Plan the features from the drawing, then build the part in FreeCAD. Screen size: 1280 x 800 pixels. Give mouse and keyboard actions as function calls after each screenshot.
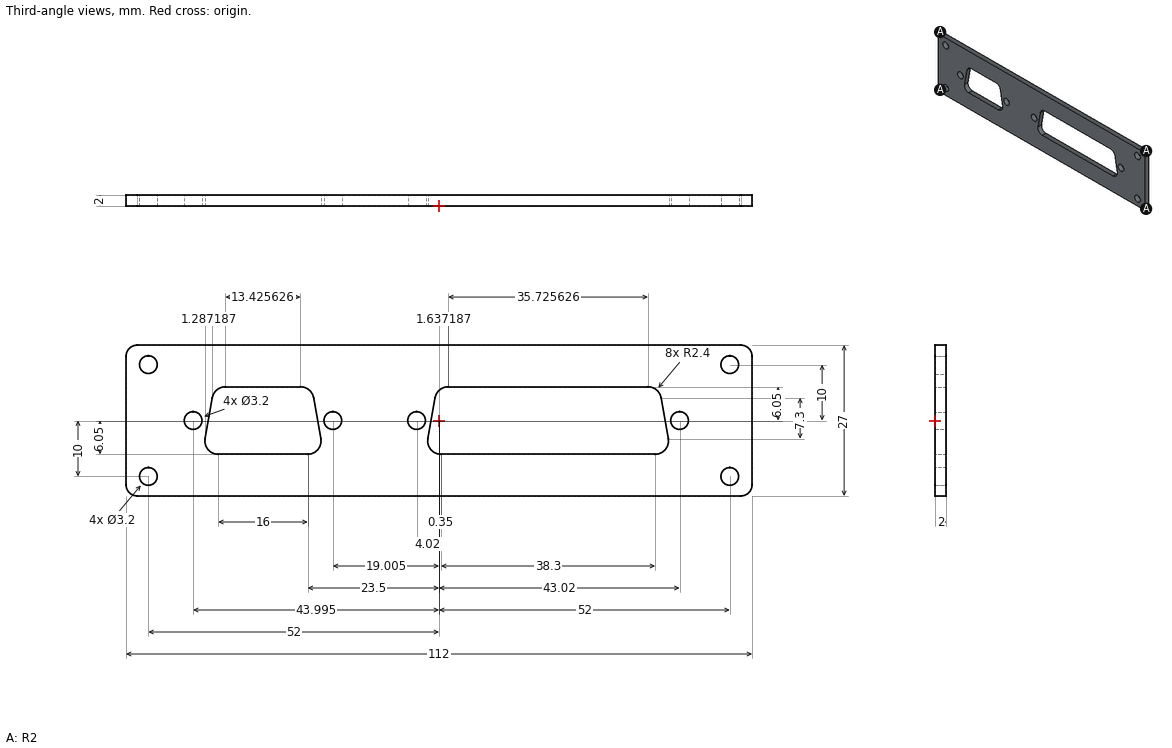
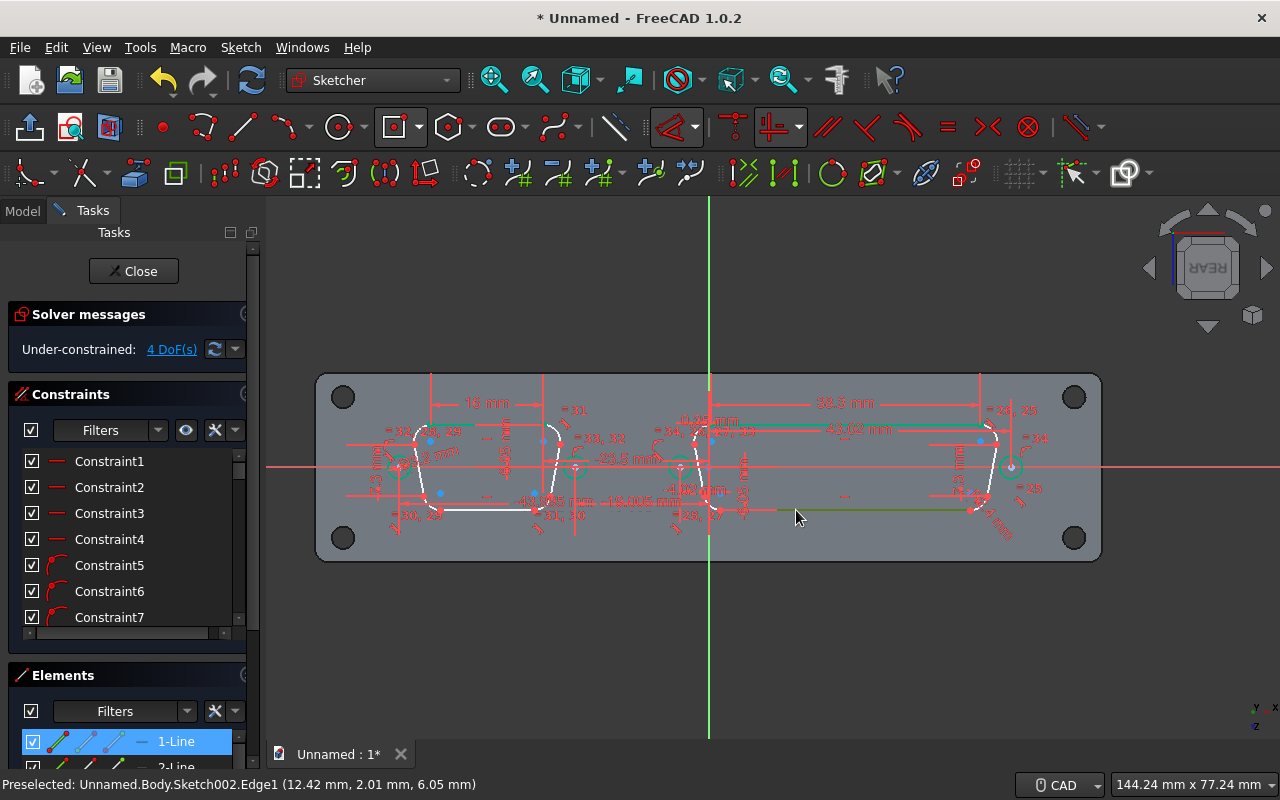
key(l)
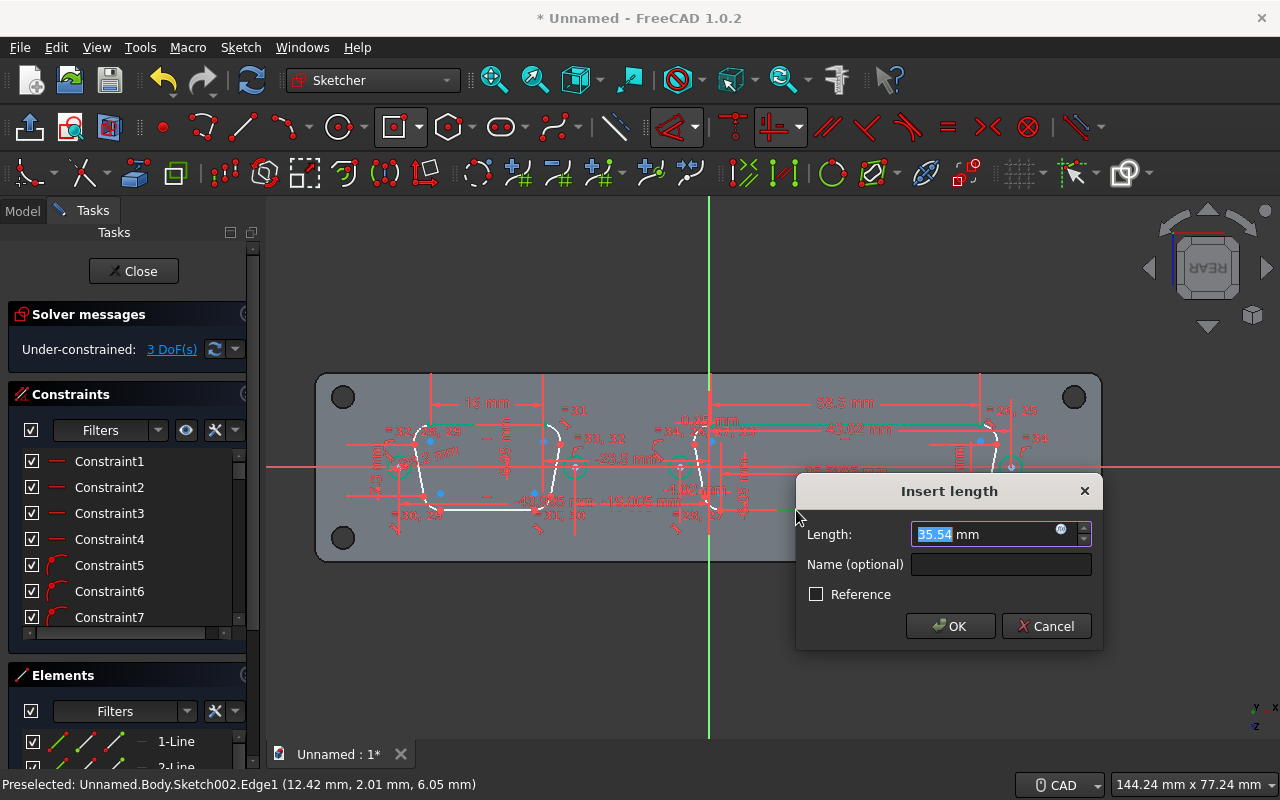
text(35.725626)
key(Return)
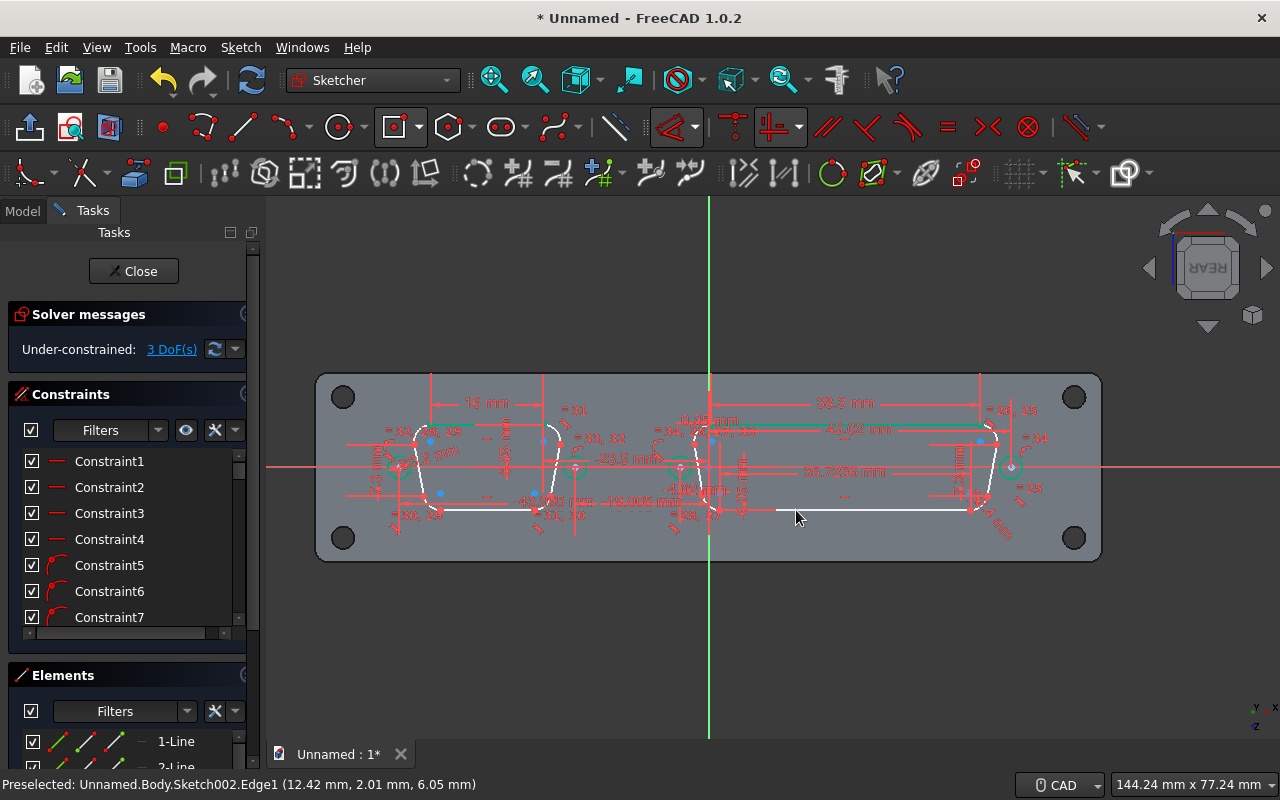
click(469, 510)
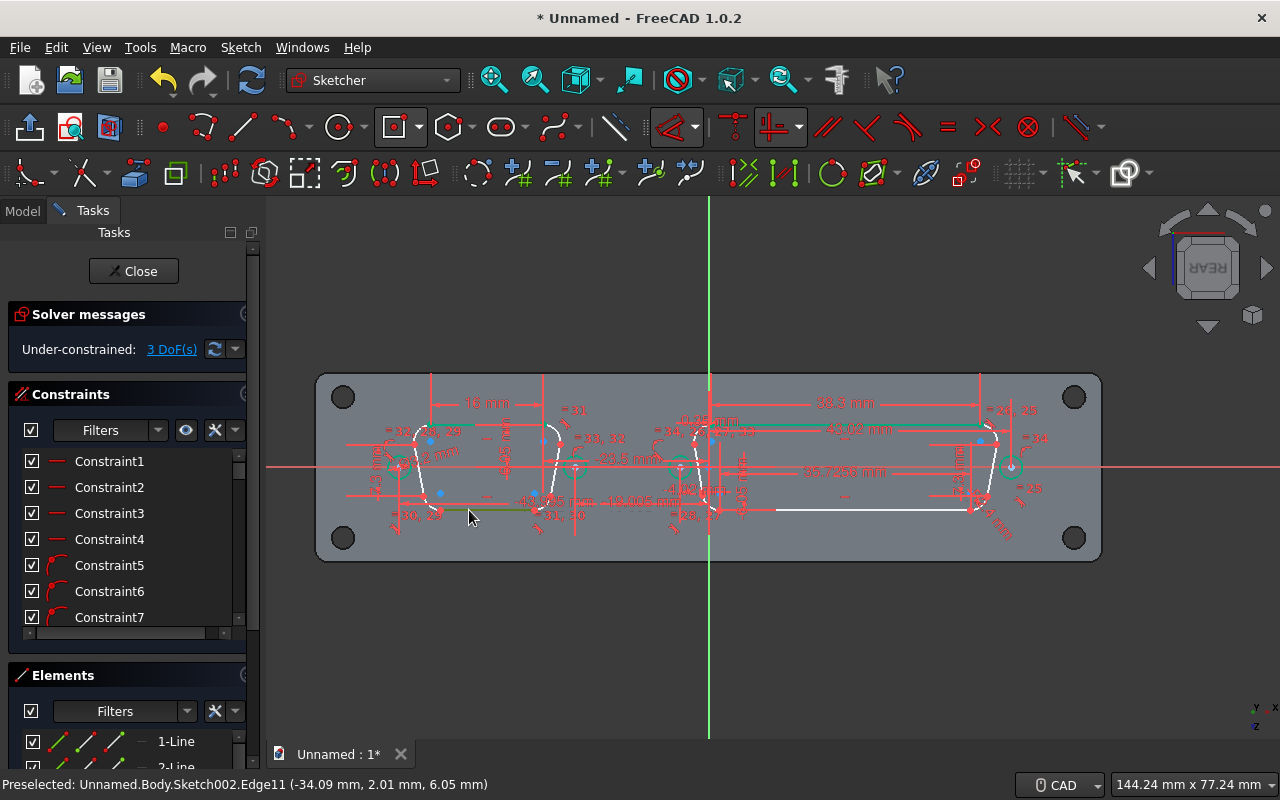
key(l)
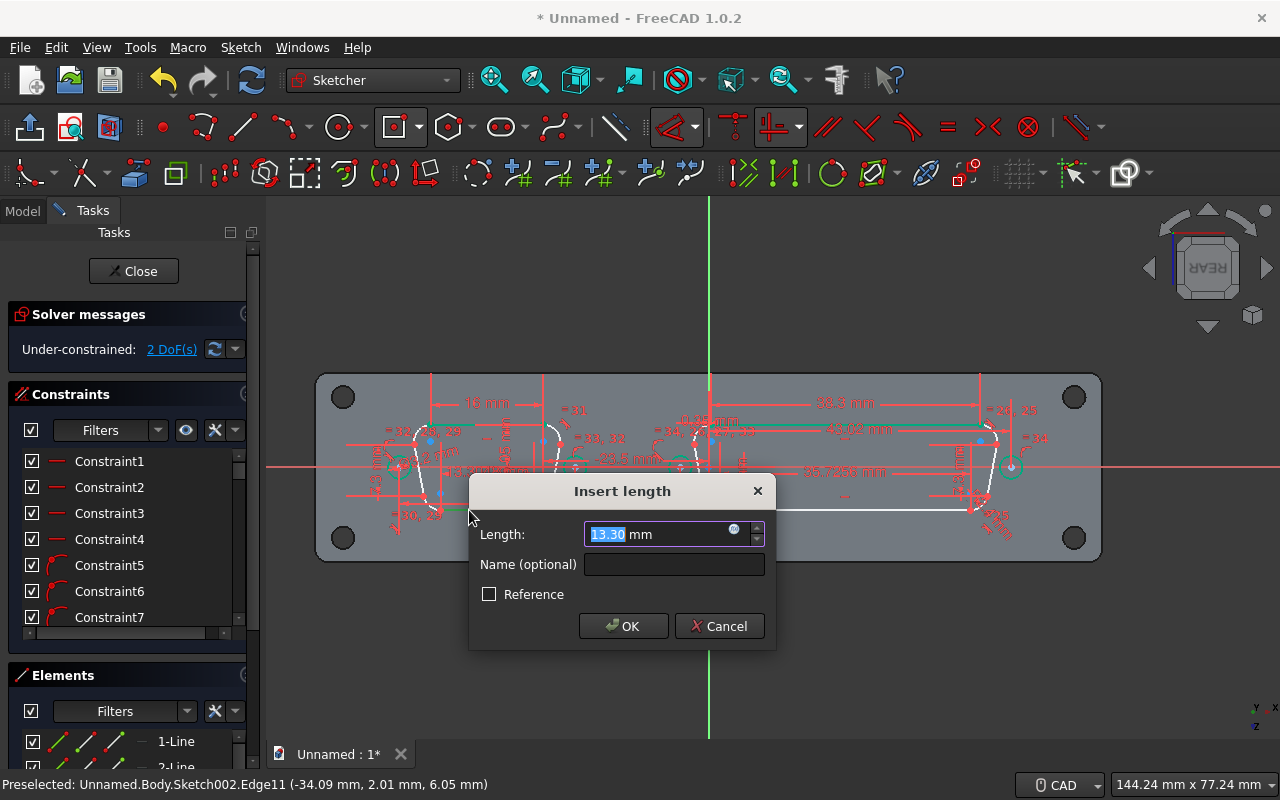
text(13.425626)
key(Return)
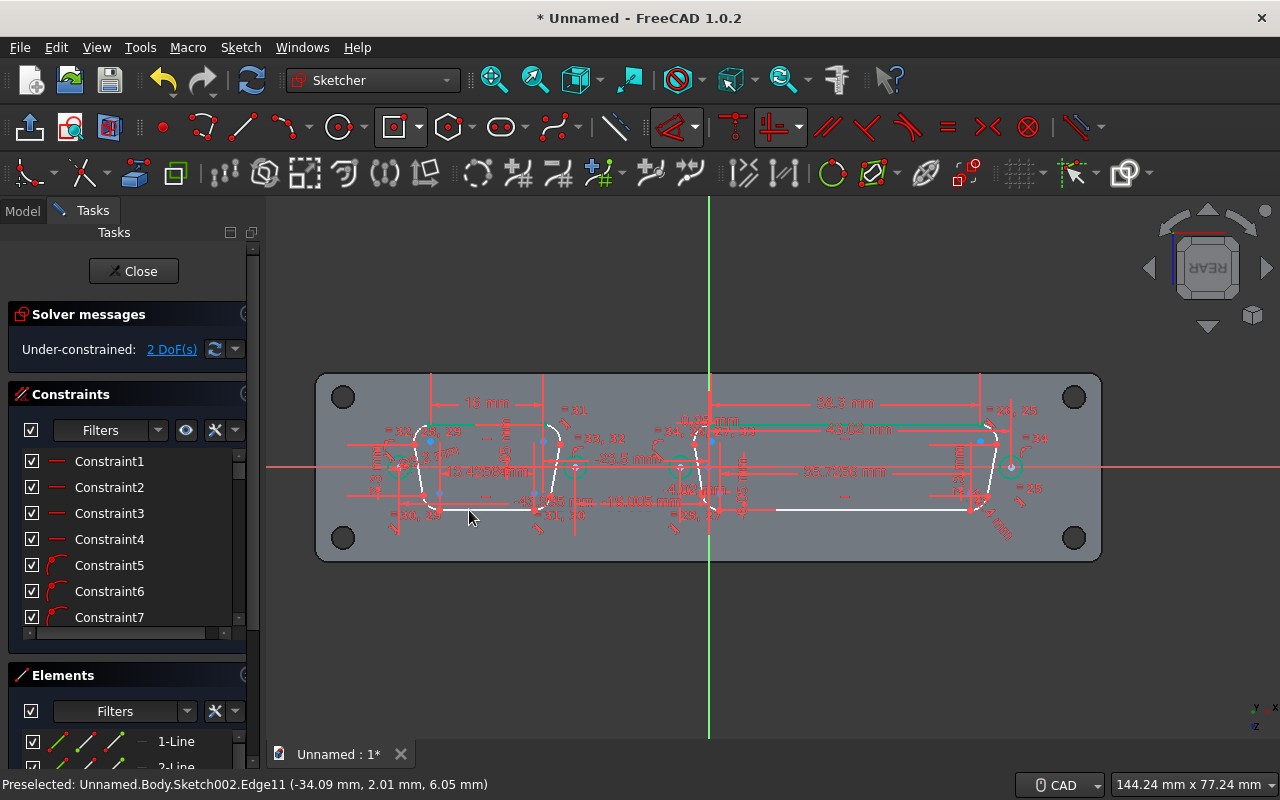
scroll(720, 510, up, 7)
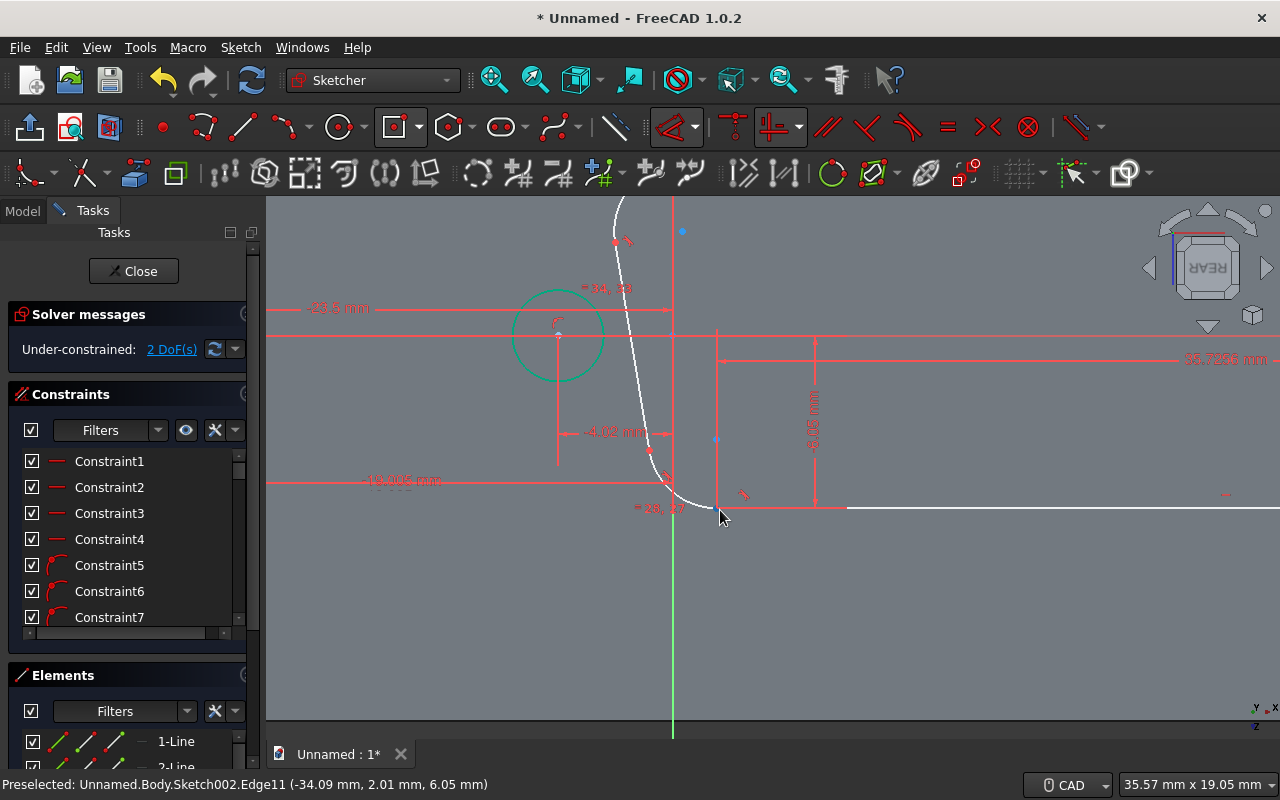
click(717, 508)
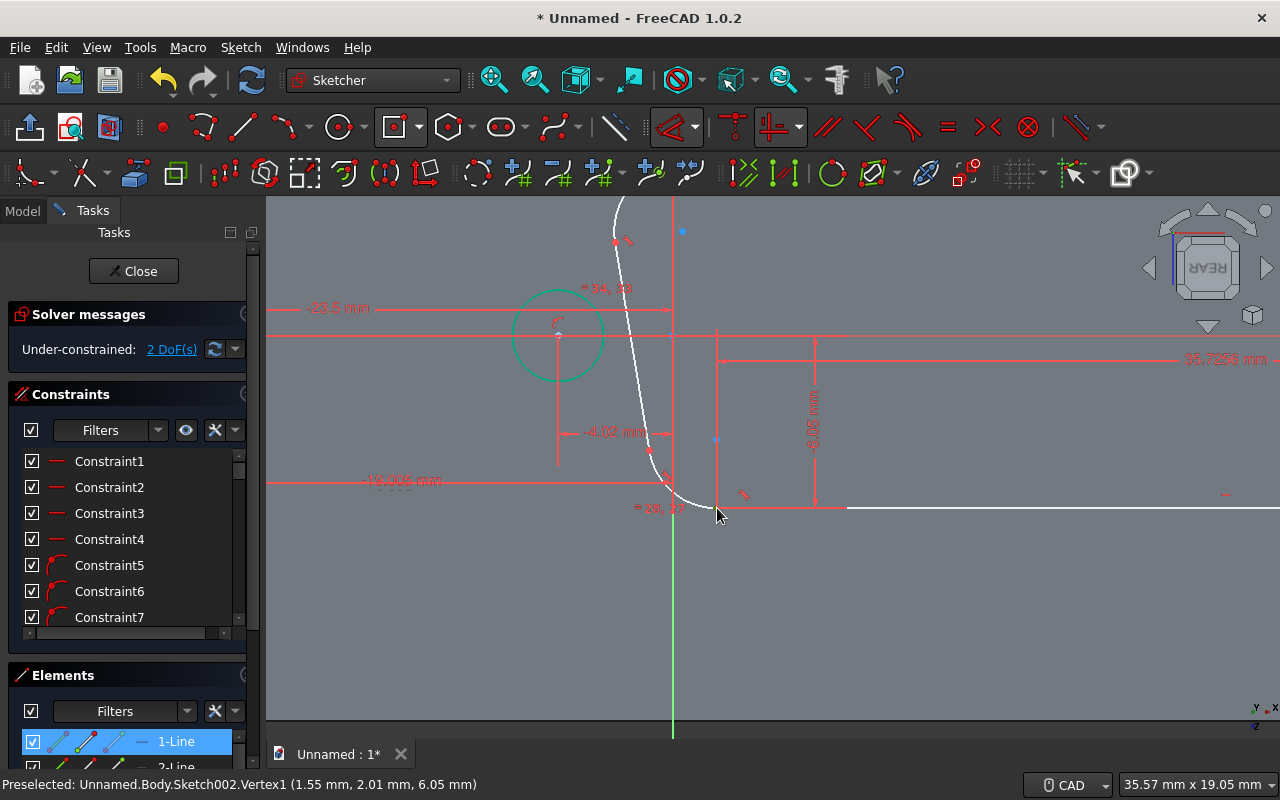
click(698, 128)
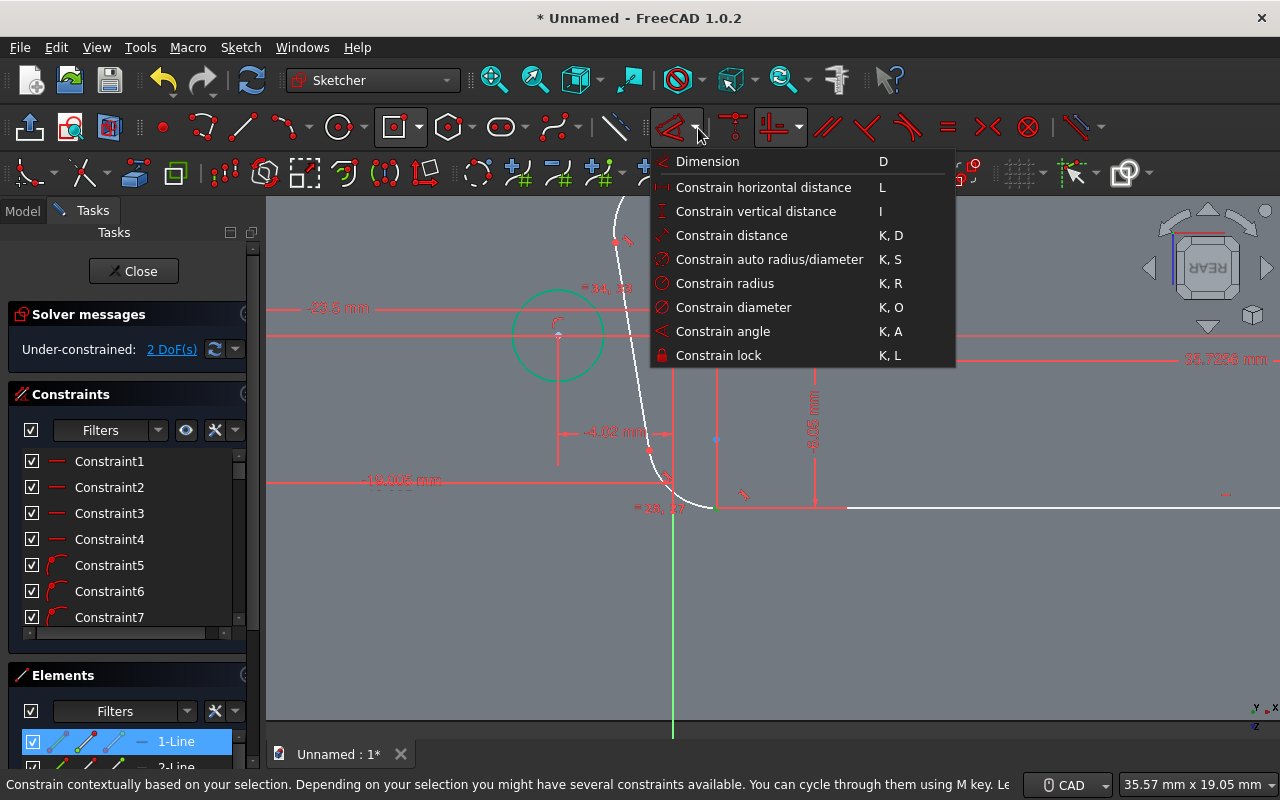
click(803, 187)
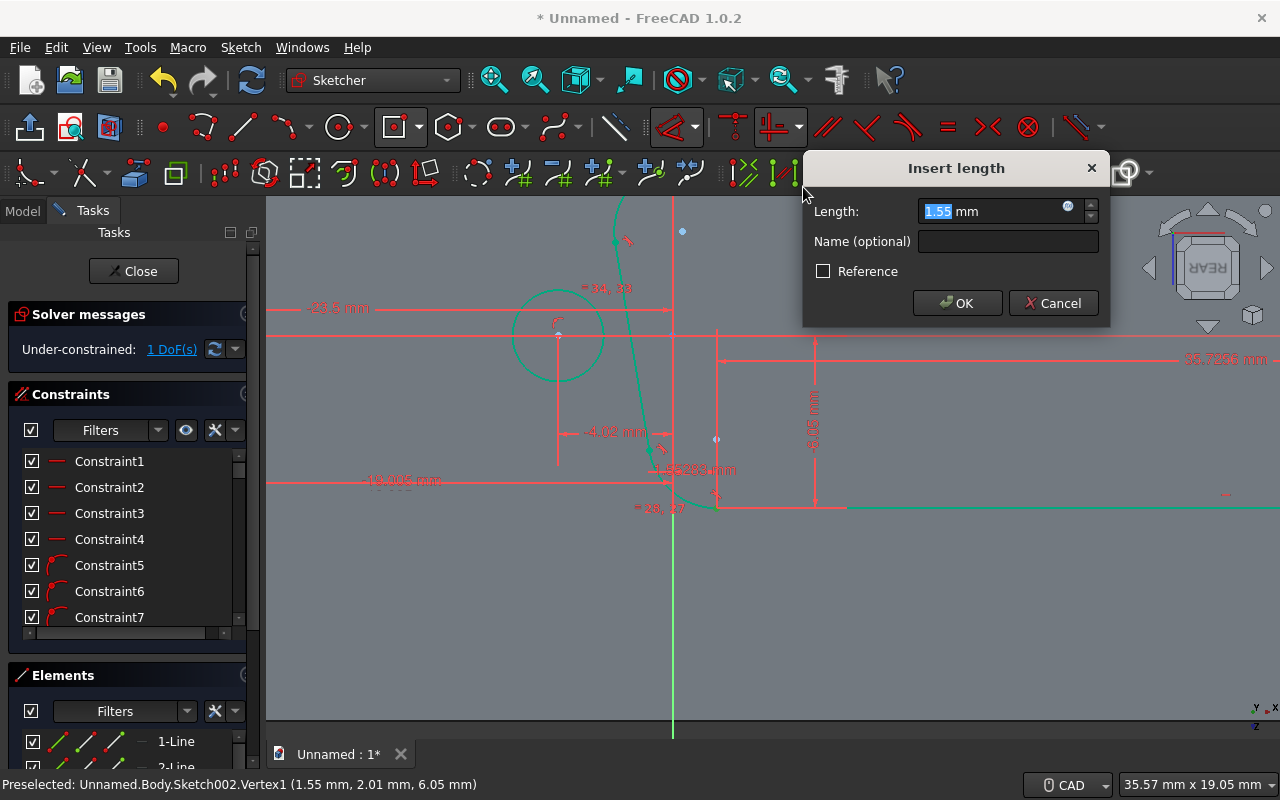
text(1.637187)
key(Return)